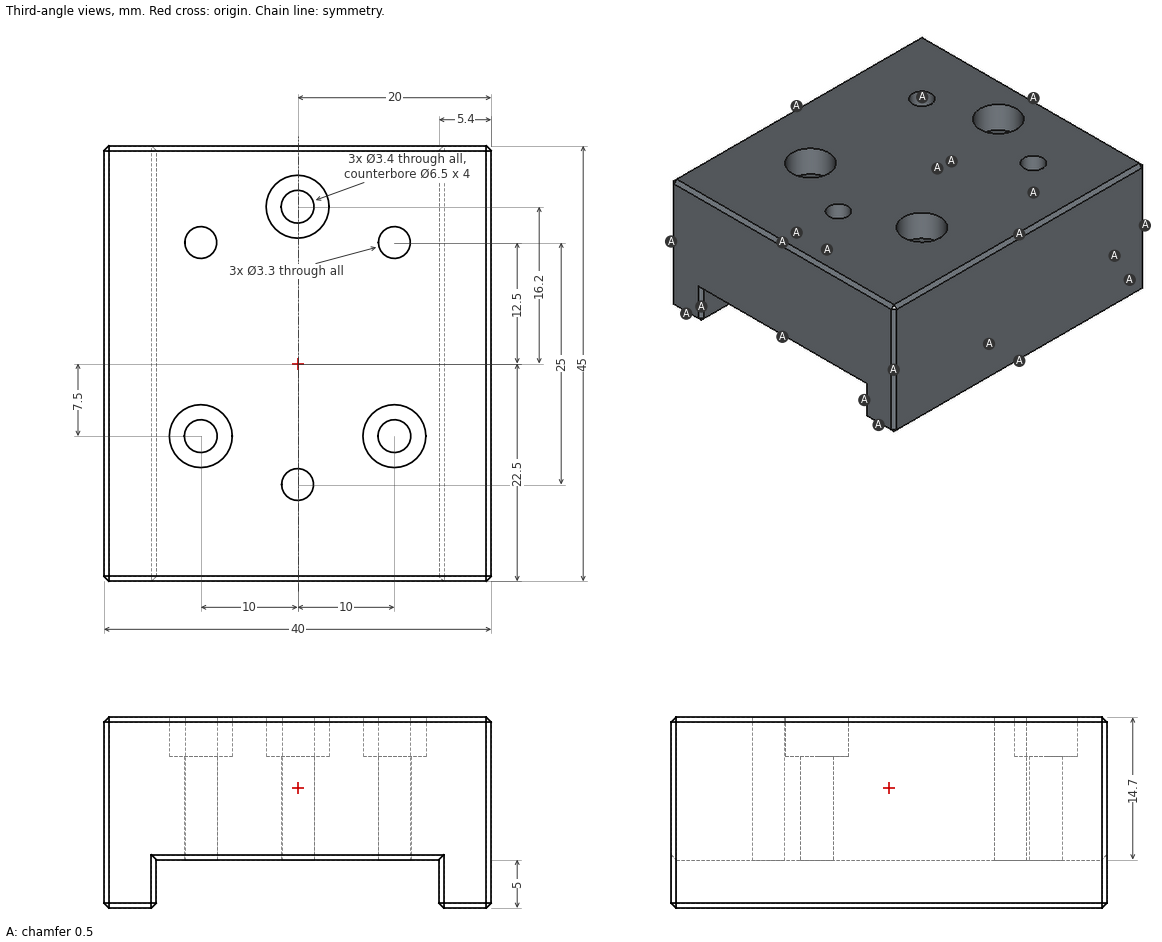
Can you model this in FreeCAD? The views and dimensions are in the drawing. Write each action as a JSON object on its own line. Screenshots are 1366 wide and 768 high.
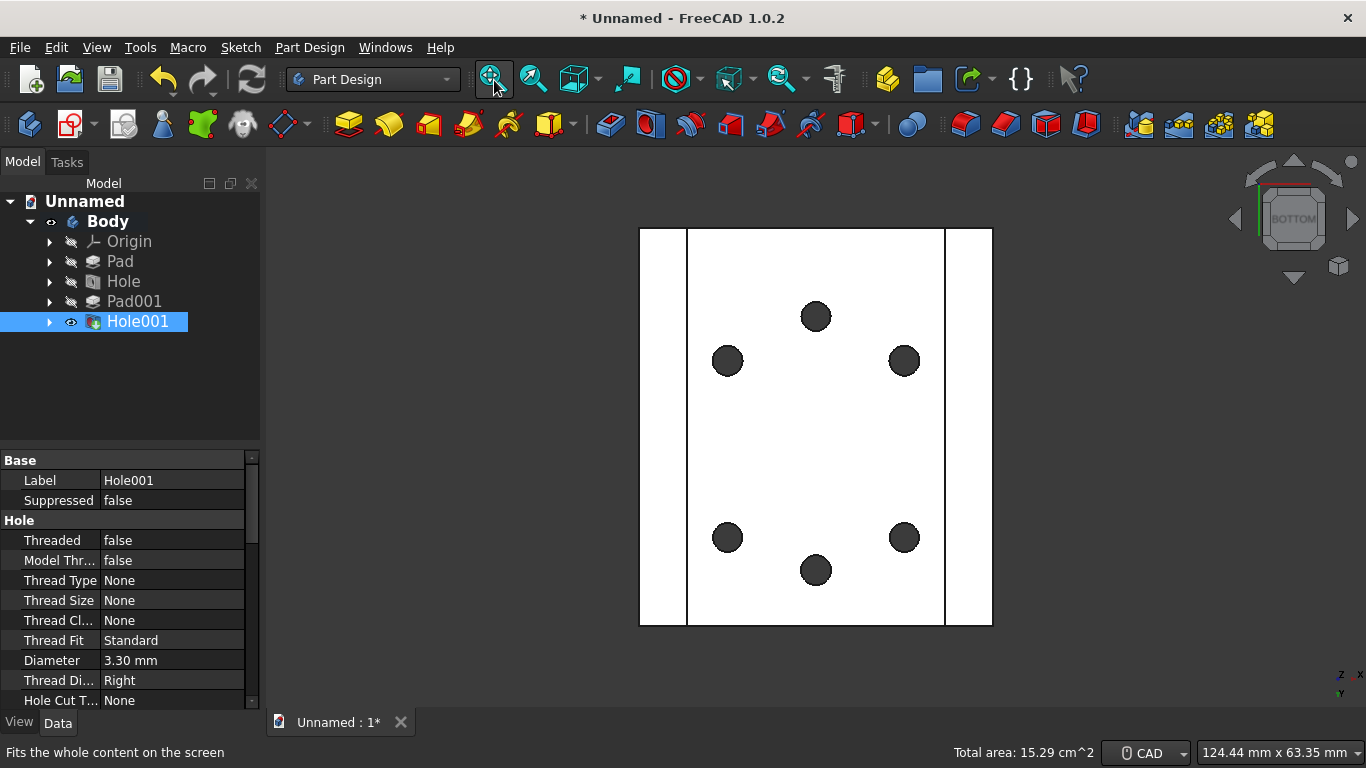
{"action": "left_click", "coordinate": [945, 426], "text": "ctrl"}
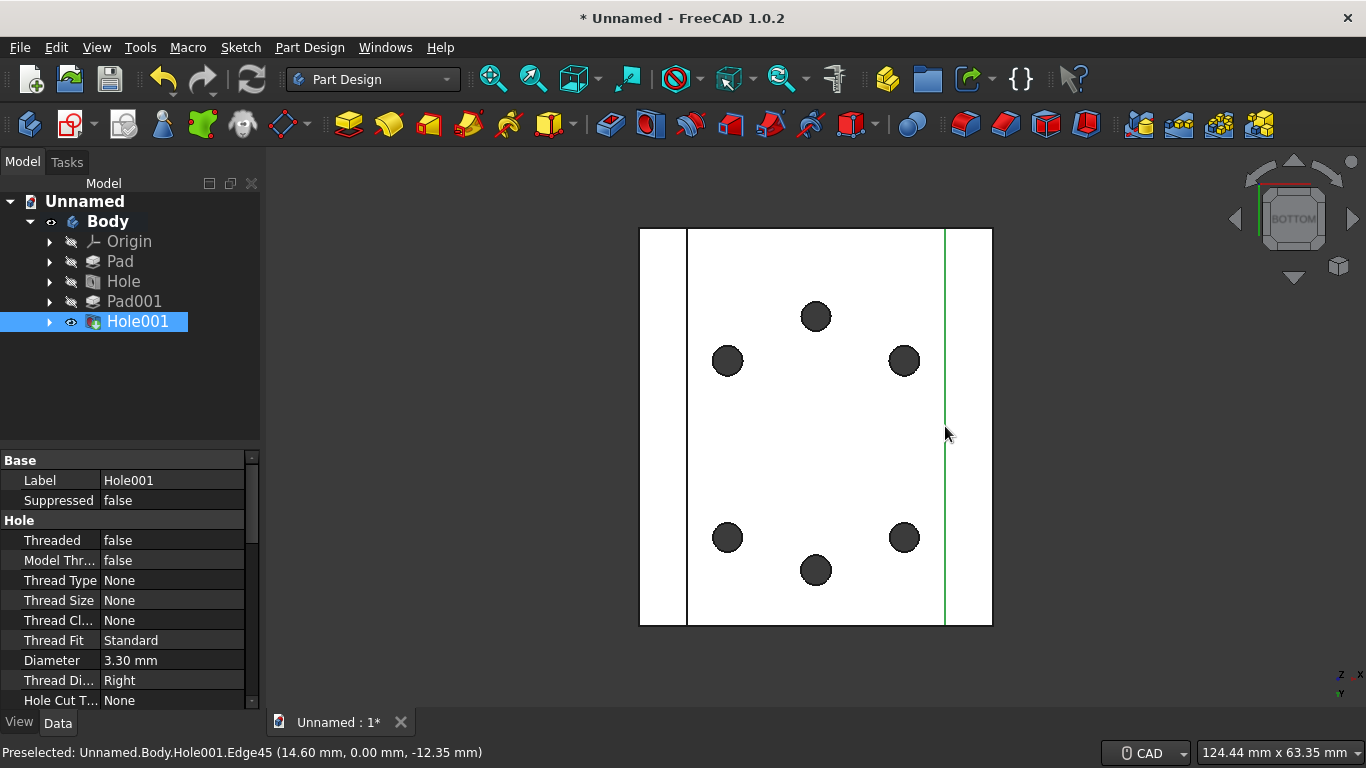
{"action": "left_click", "coordinate": [687, 426], "text": "ctrl"}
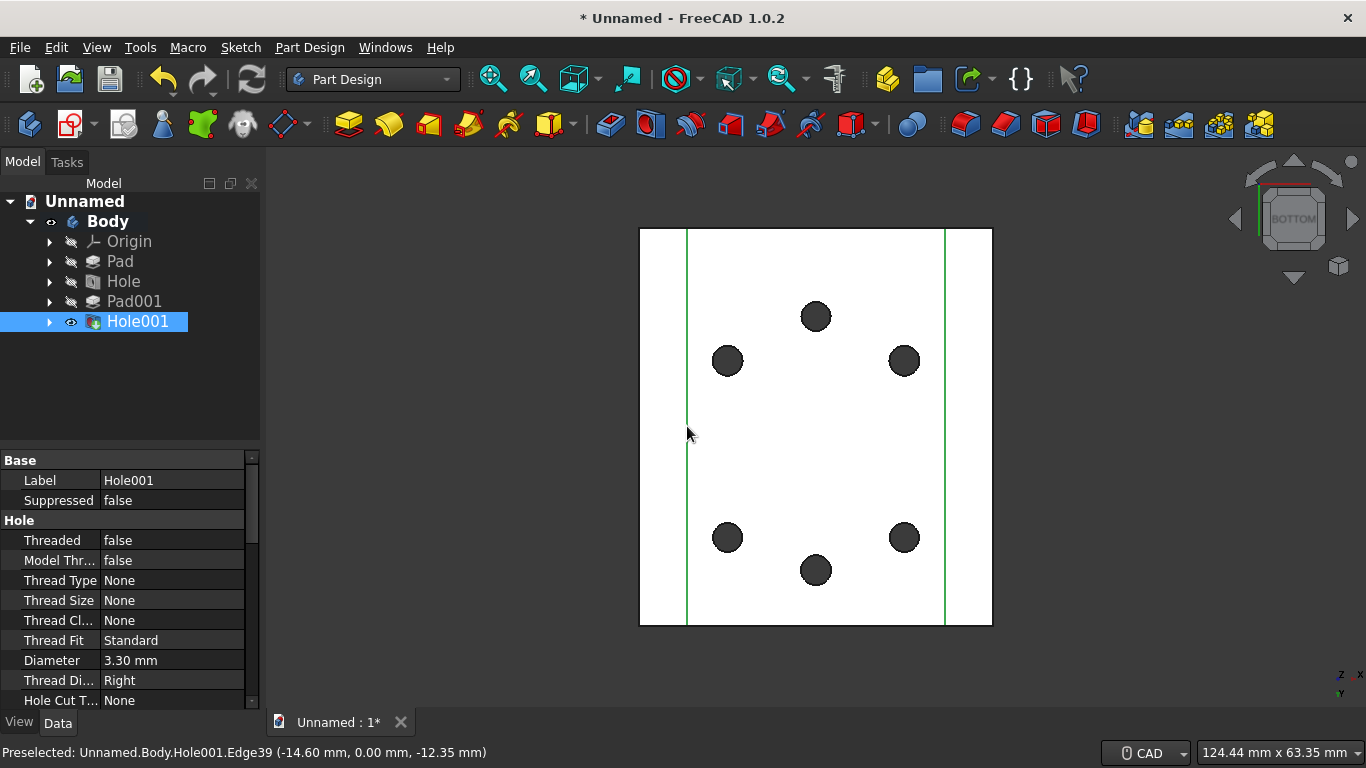
{"action": "key", "text": "4"}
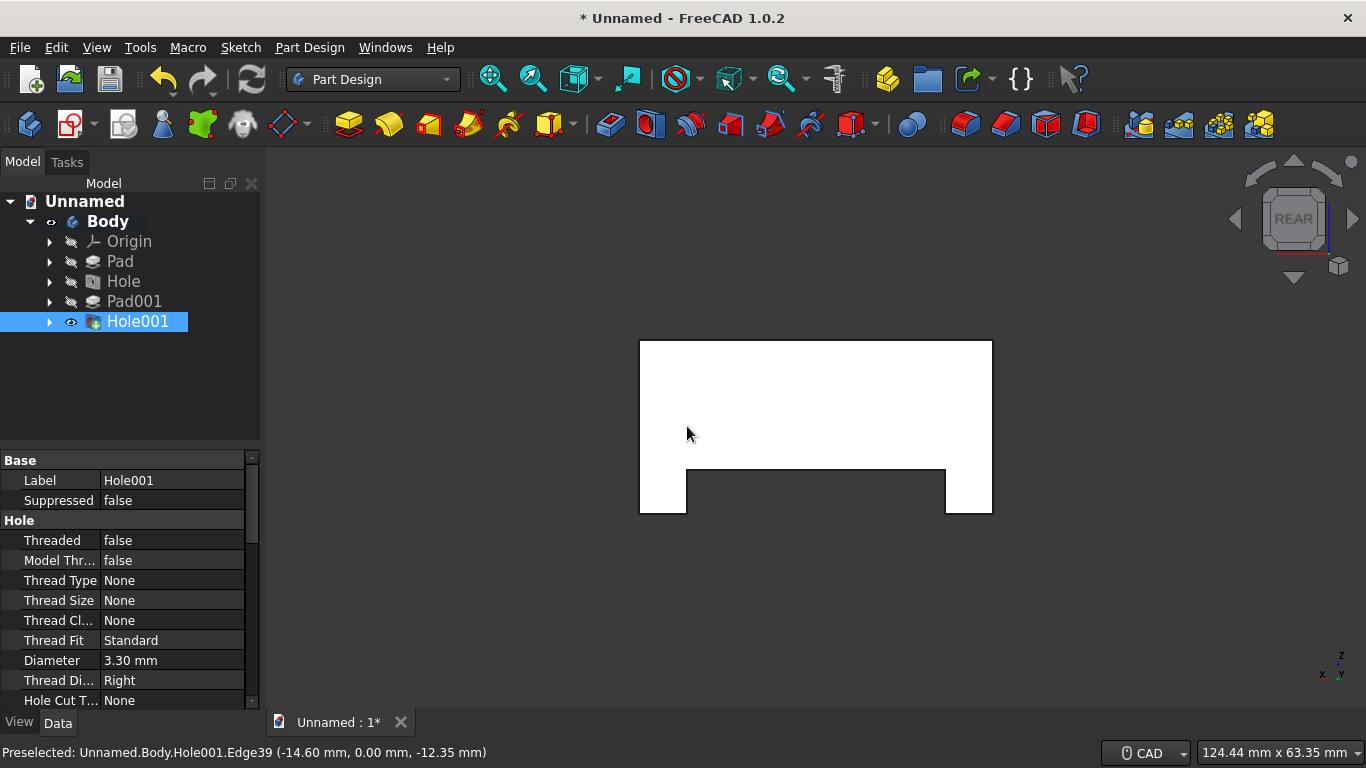
{"action": "left_click", "coordinate": [494, 80]}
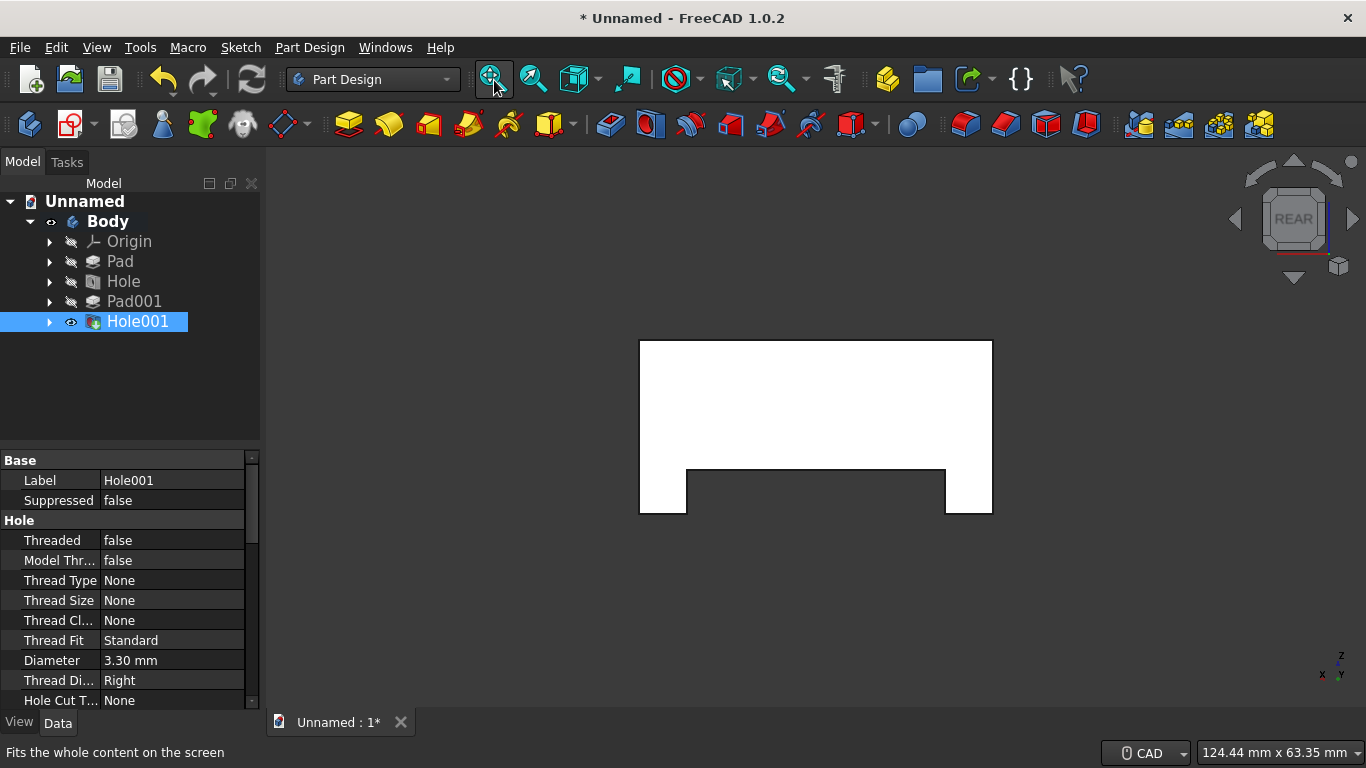
{"action": "left_click", "coordinate": [715, 401], "text": "ctrl"}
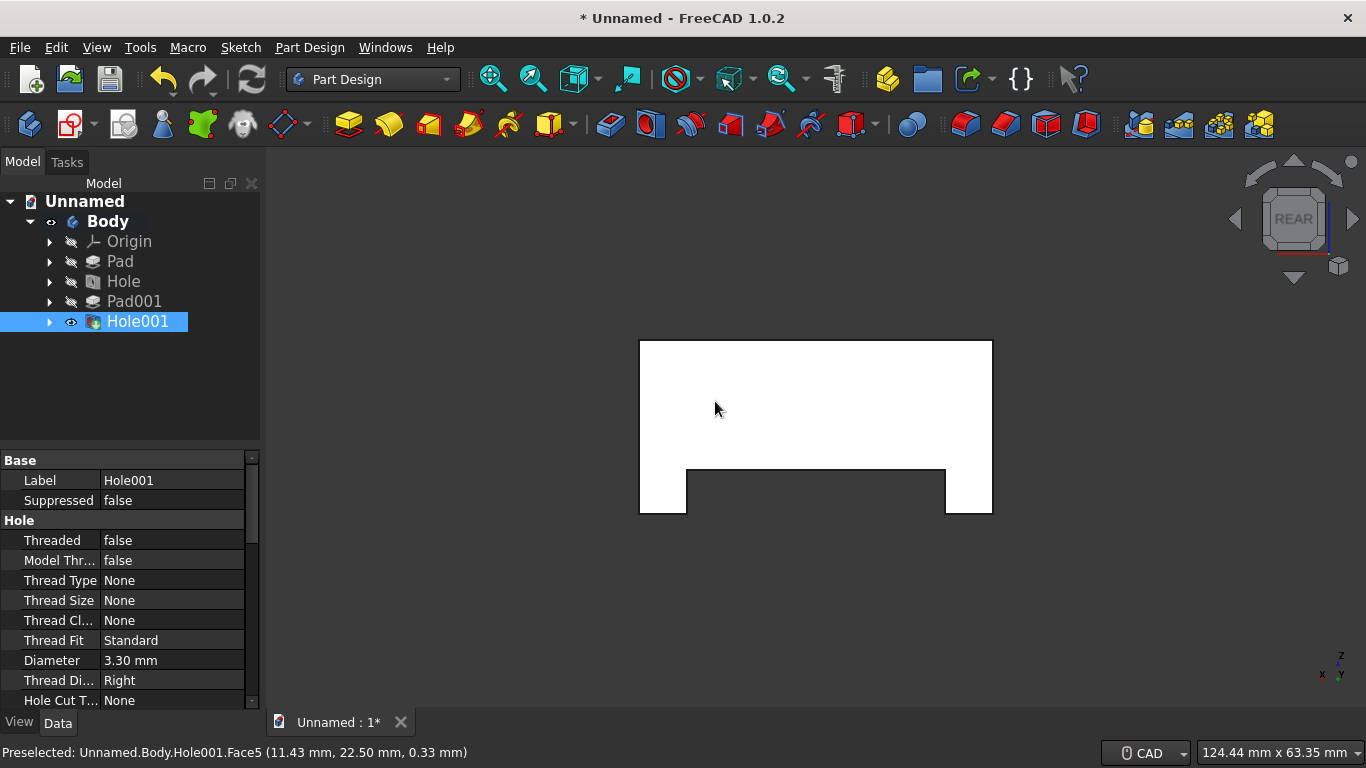
{"action": "key", "text": "6"}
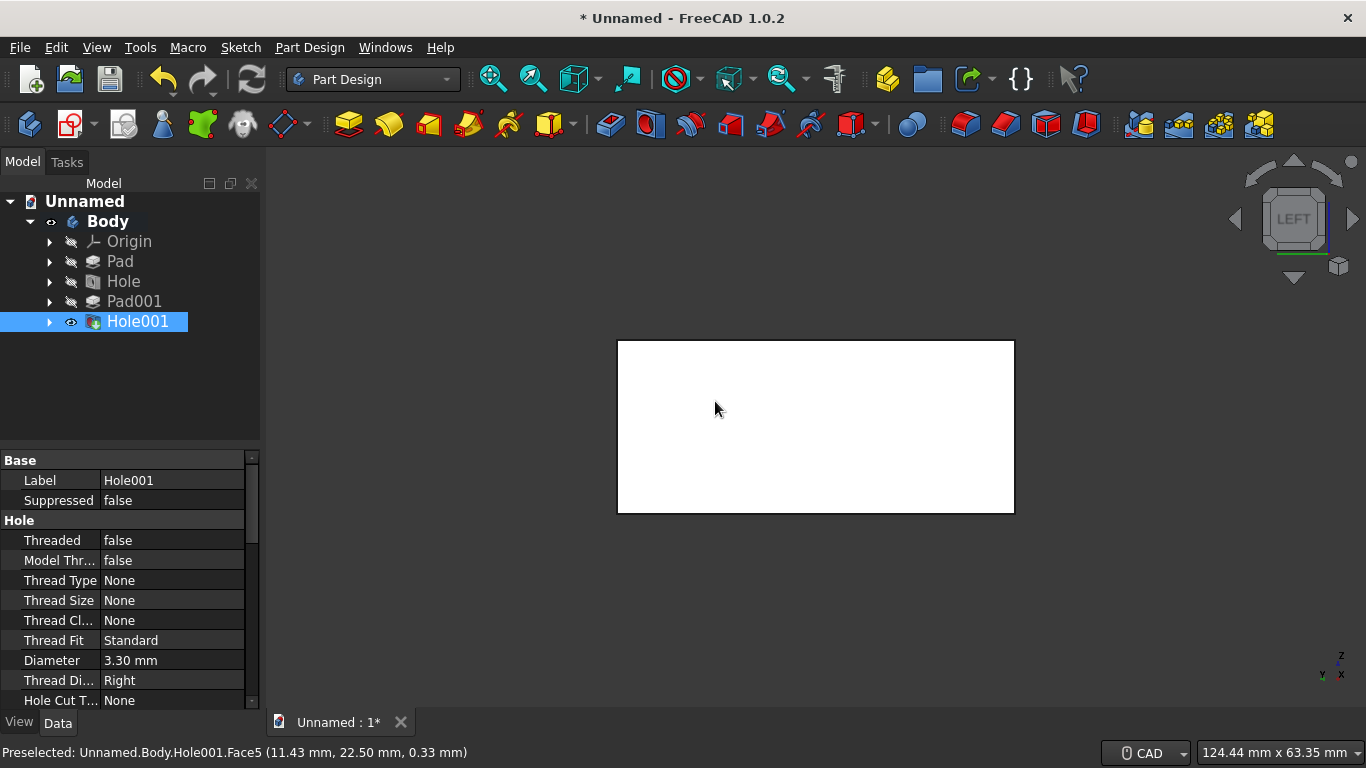
{"action": "left_click", "coordinate": [494, 80]}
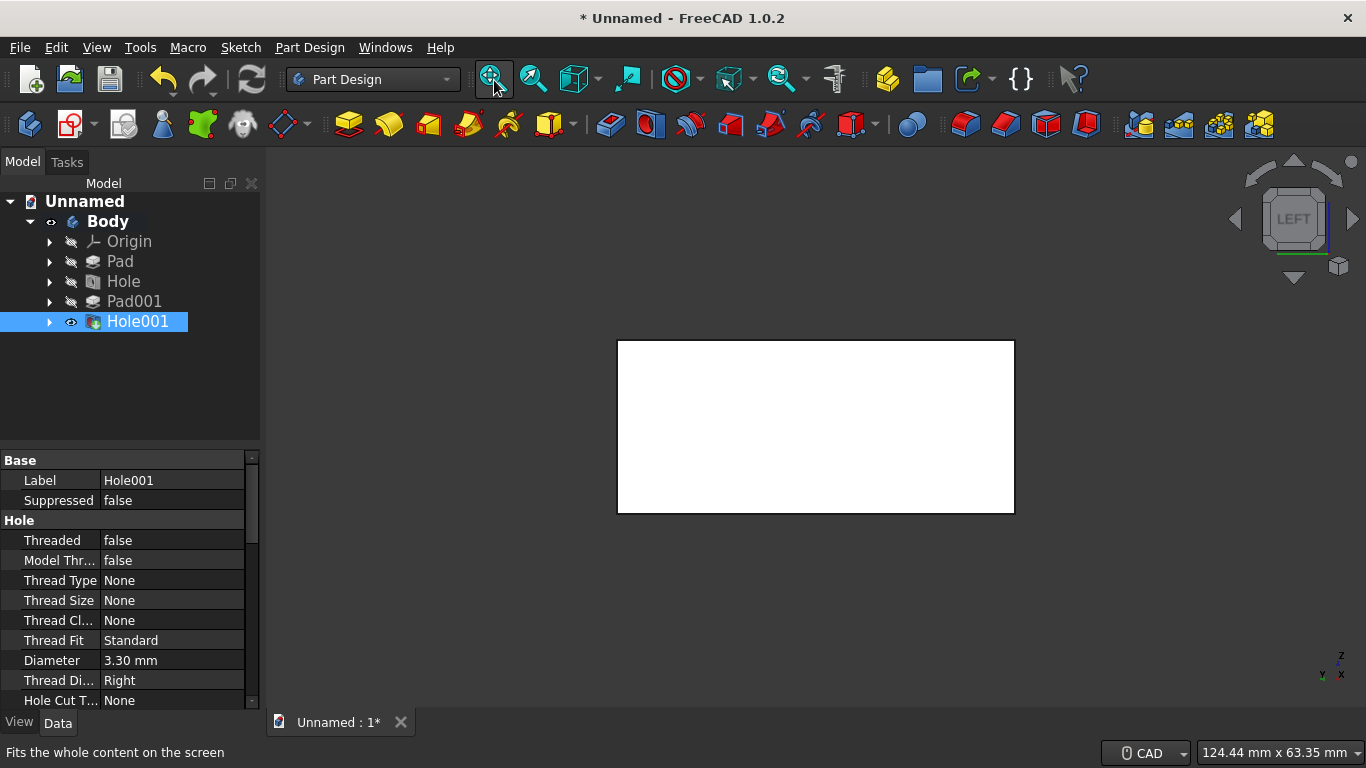
{"action": "left_click", "coordinate": [759, 426], "text": "ctrl"}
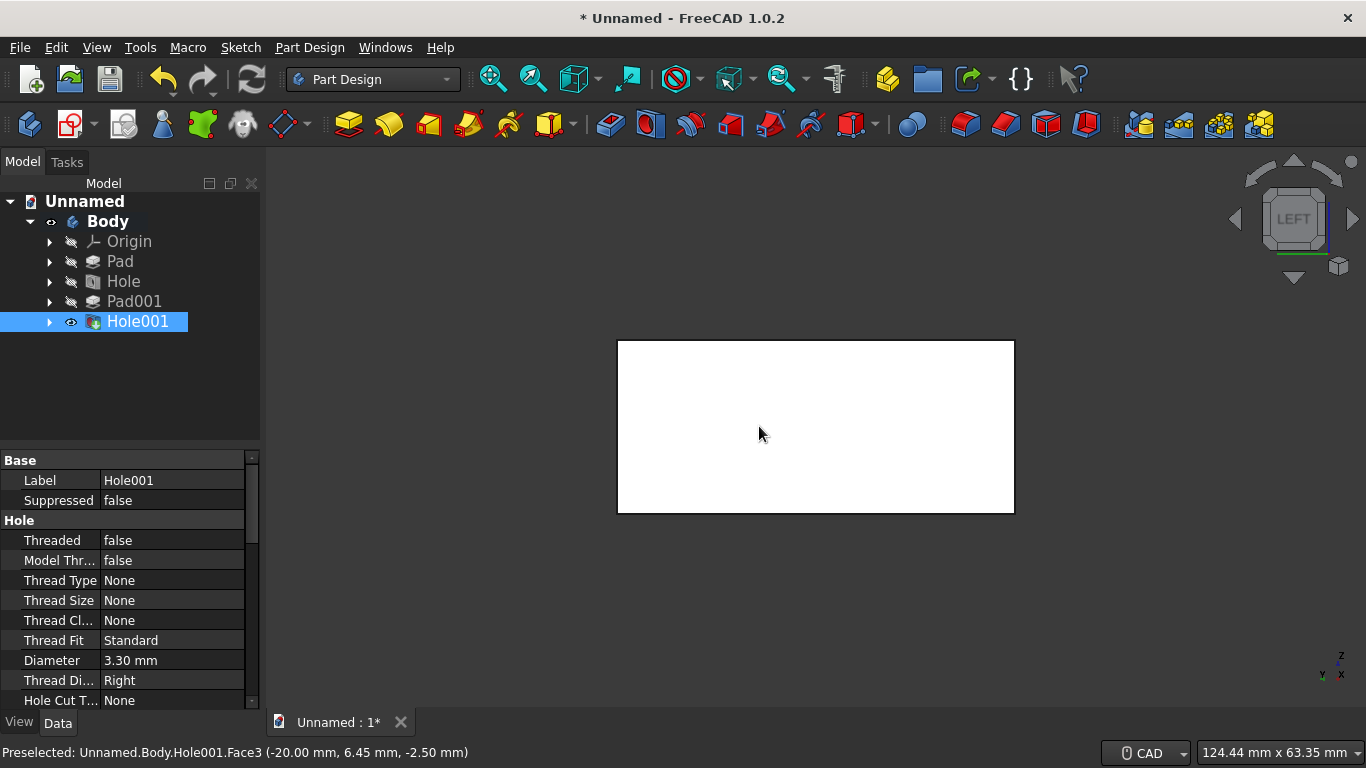
{"action": "left_click", "coordinate": [1006, 124]}